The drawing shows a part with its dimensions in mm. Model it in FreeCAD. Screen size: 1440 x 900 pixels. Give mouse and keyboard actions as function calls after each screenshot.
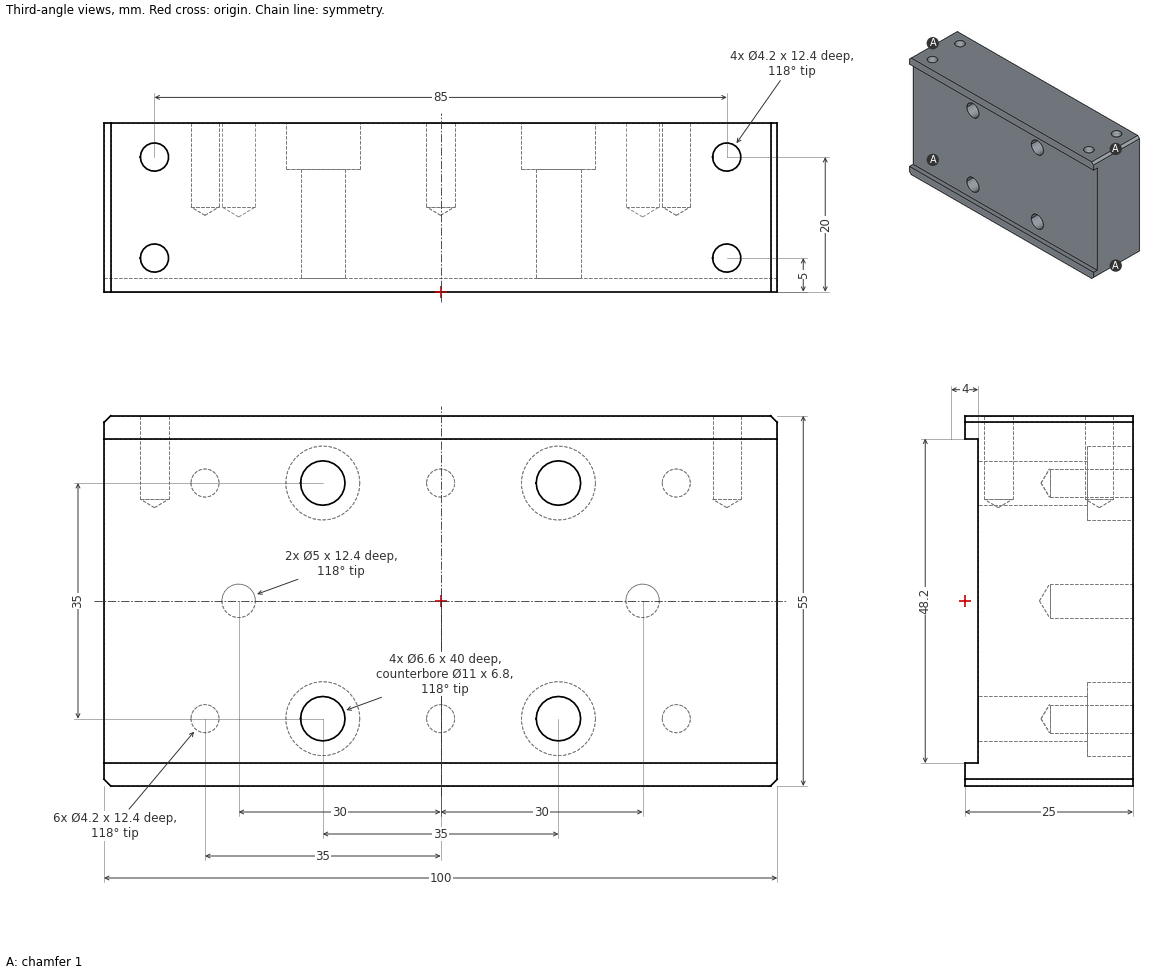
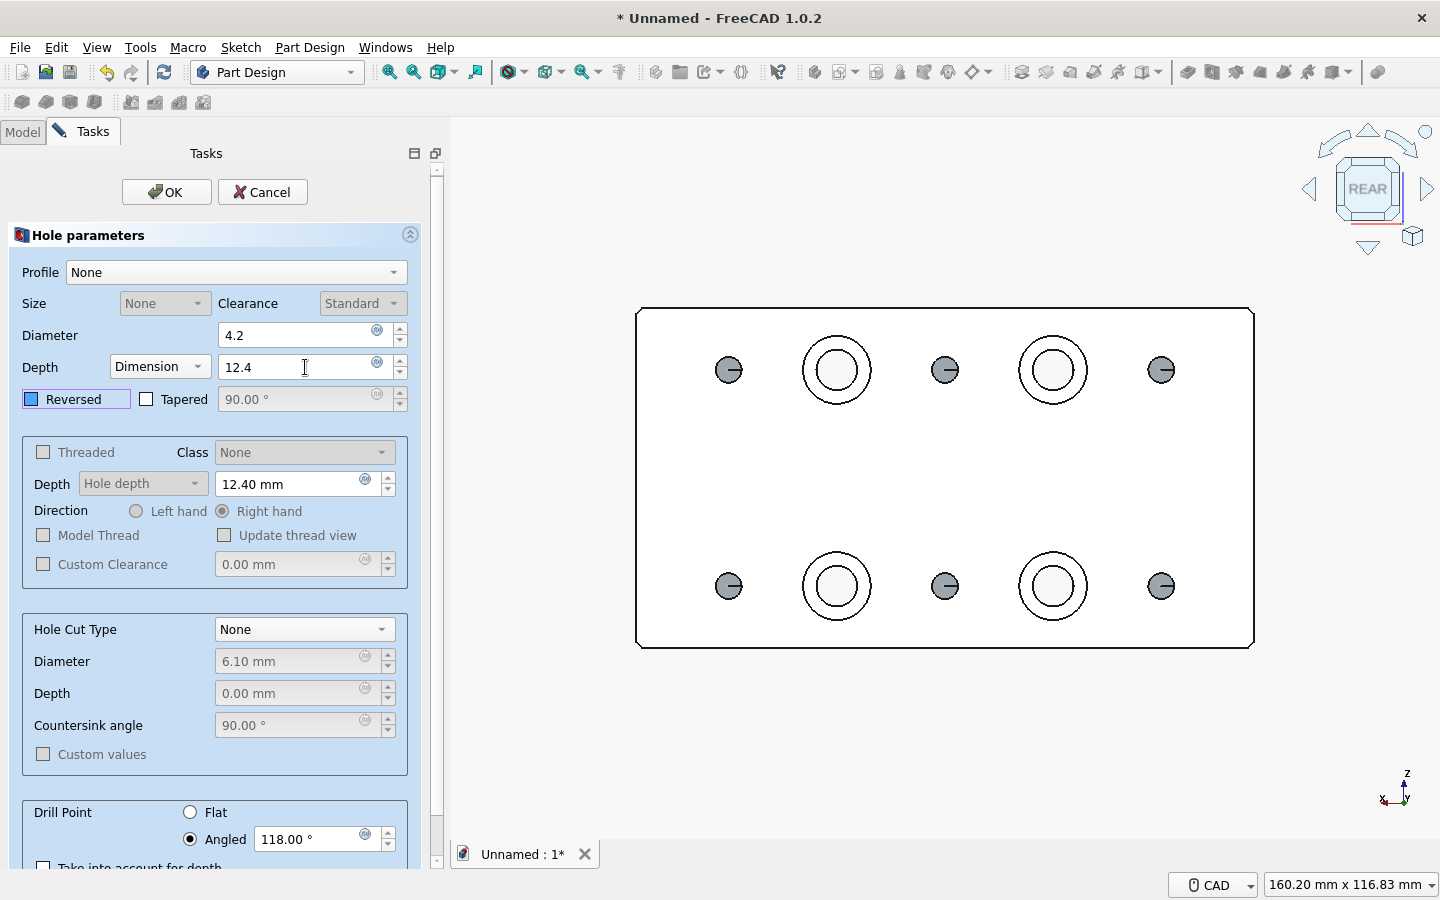
click(167, 192)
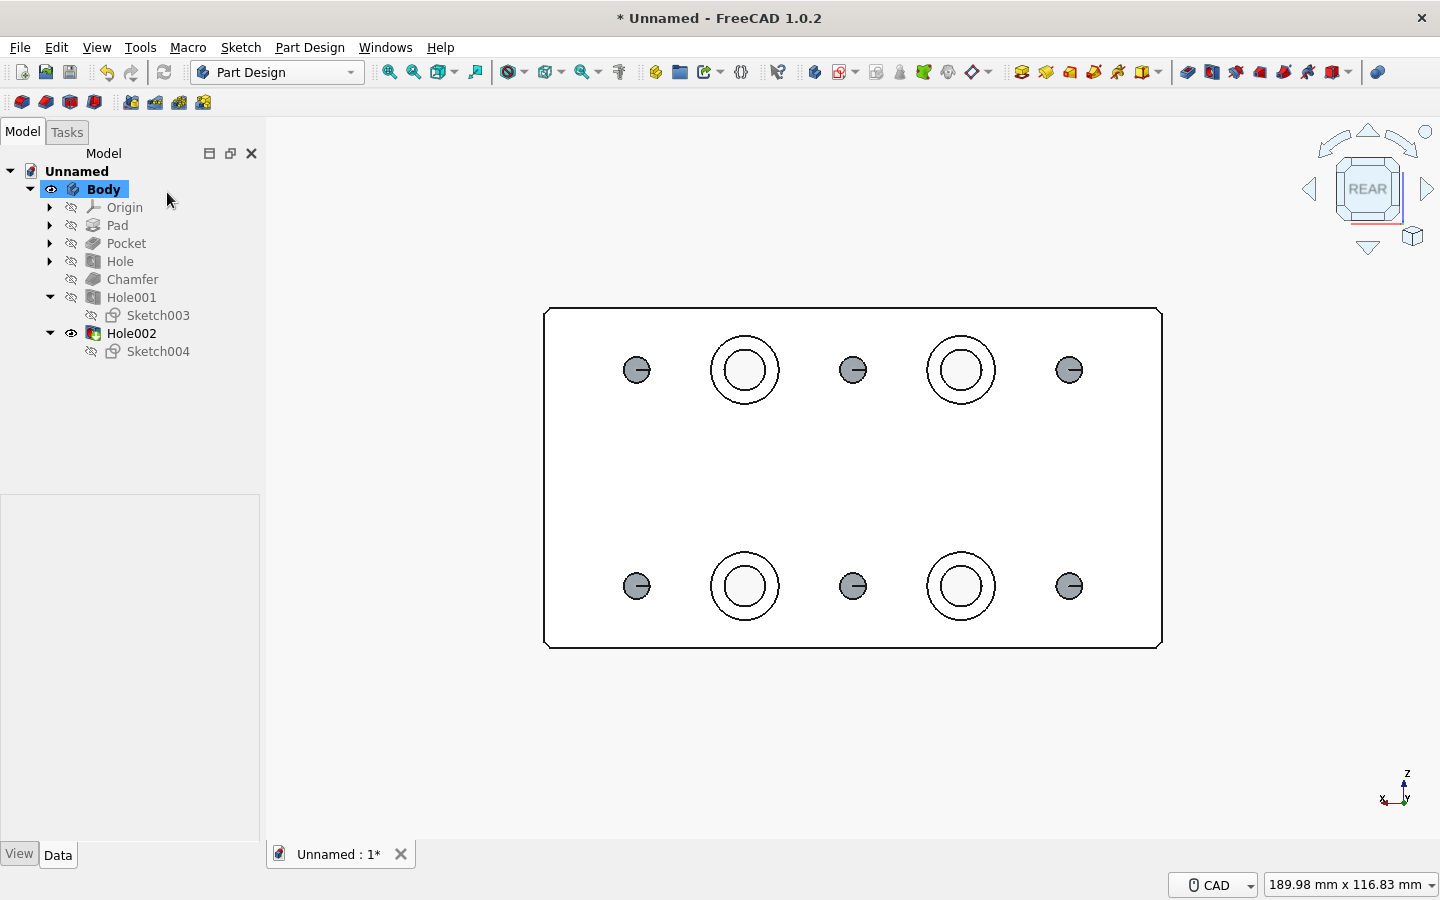
click(853, 477)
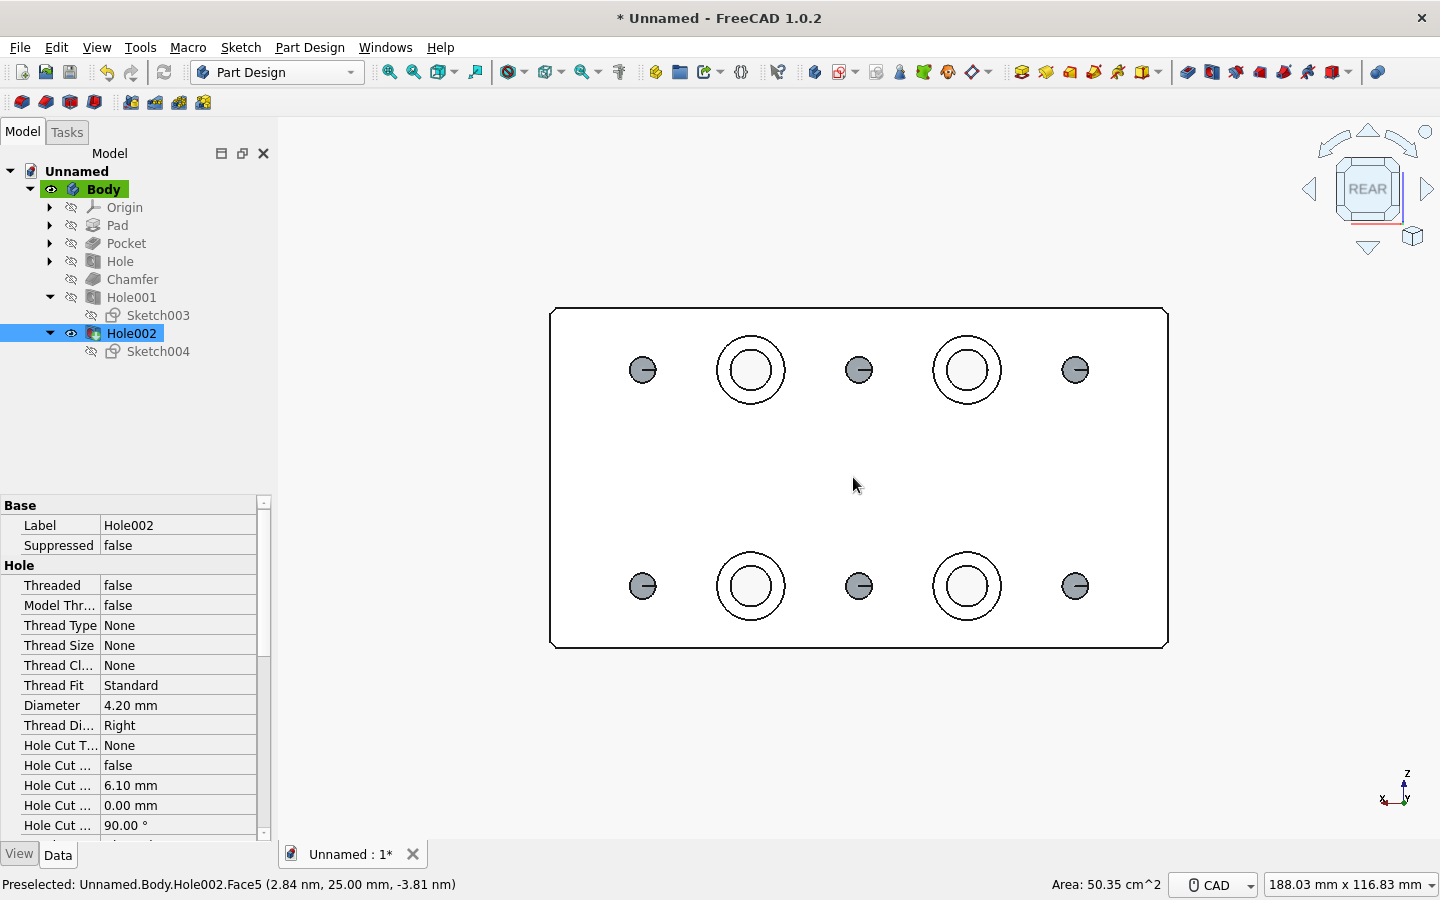
click(840, 72)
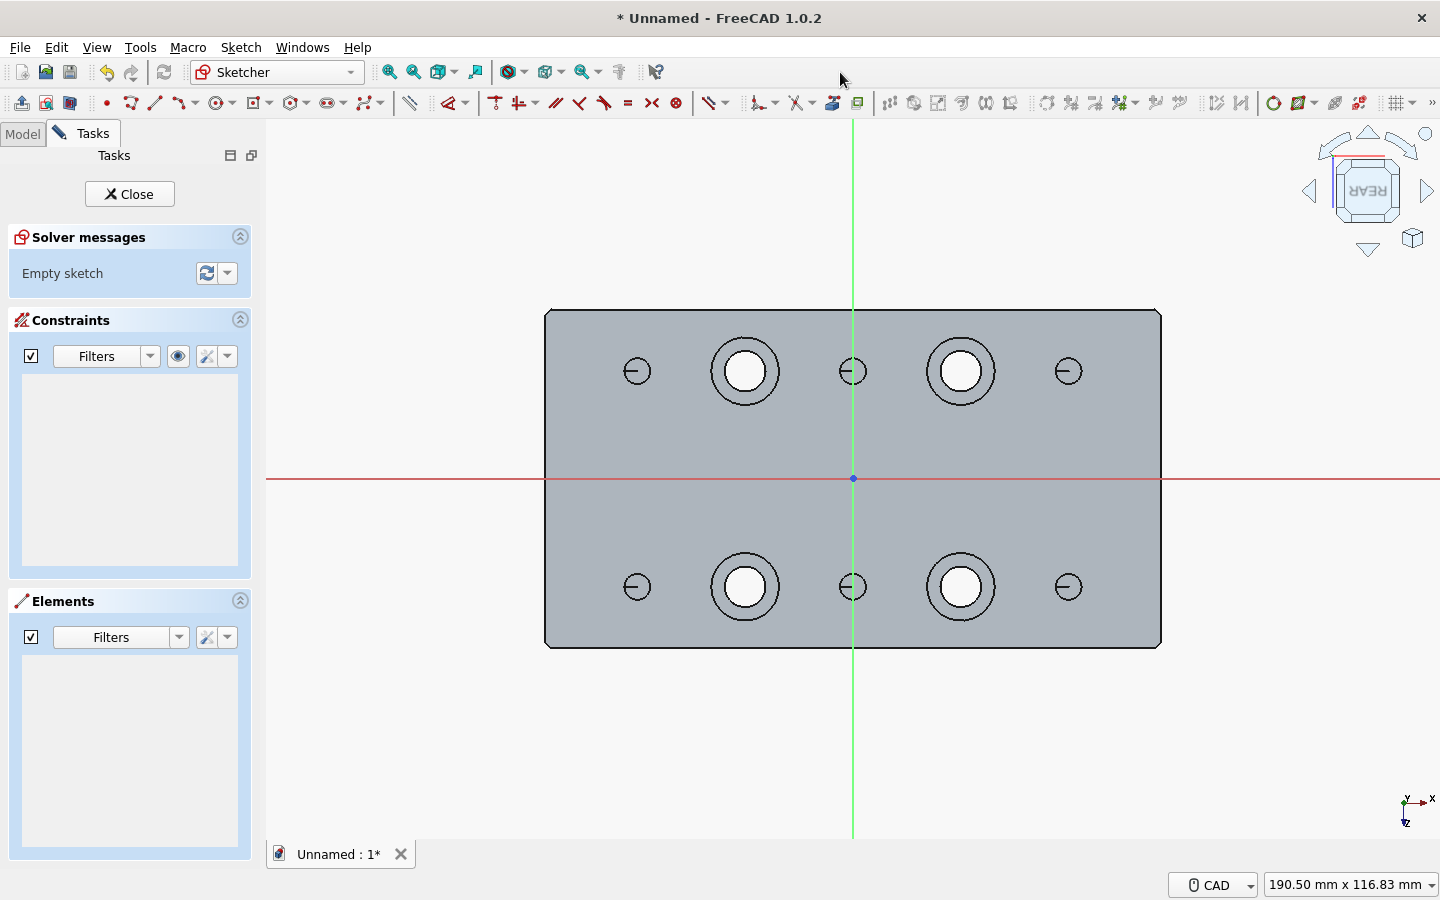
scroll(936, 479, up, 3)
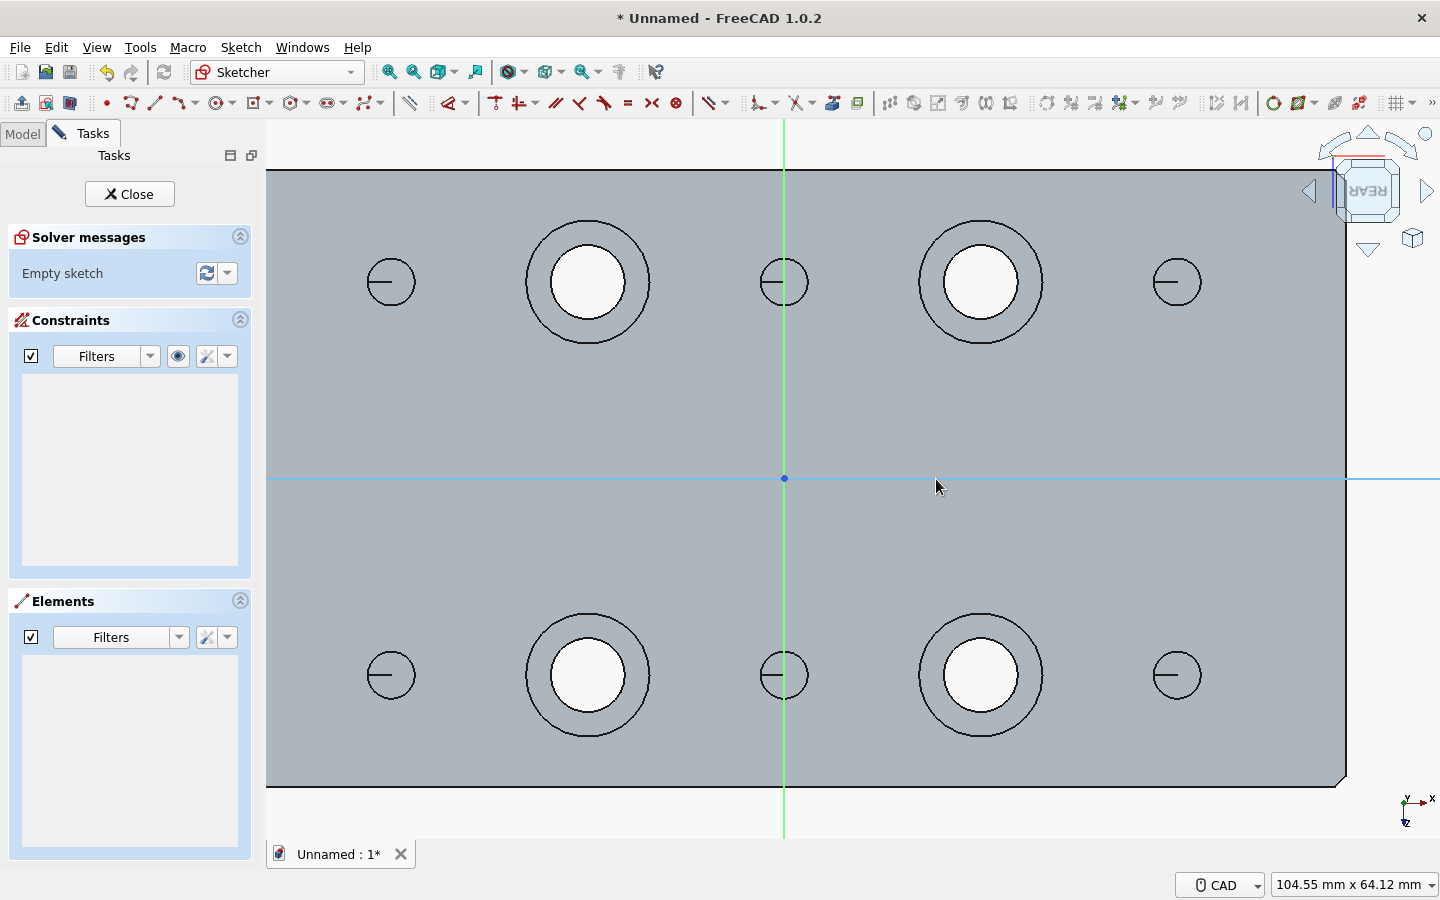
click(216, 104)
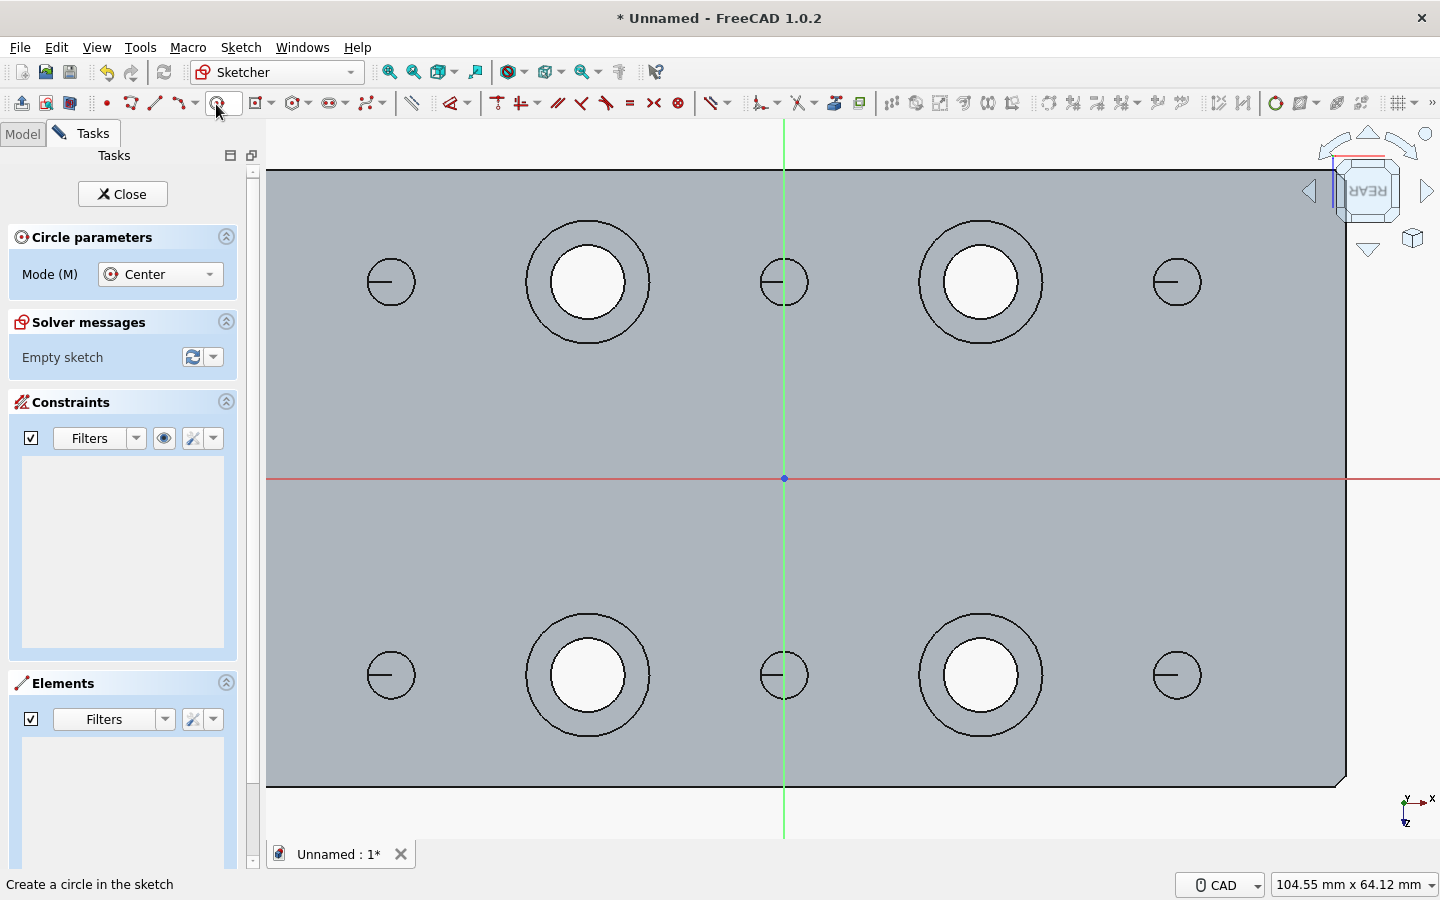
click(447, 479)
move(467, 459)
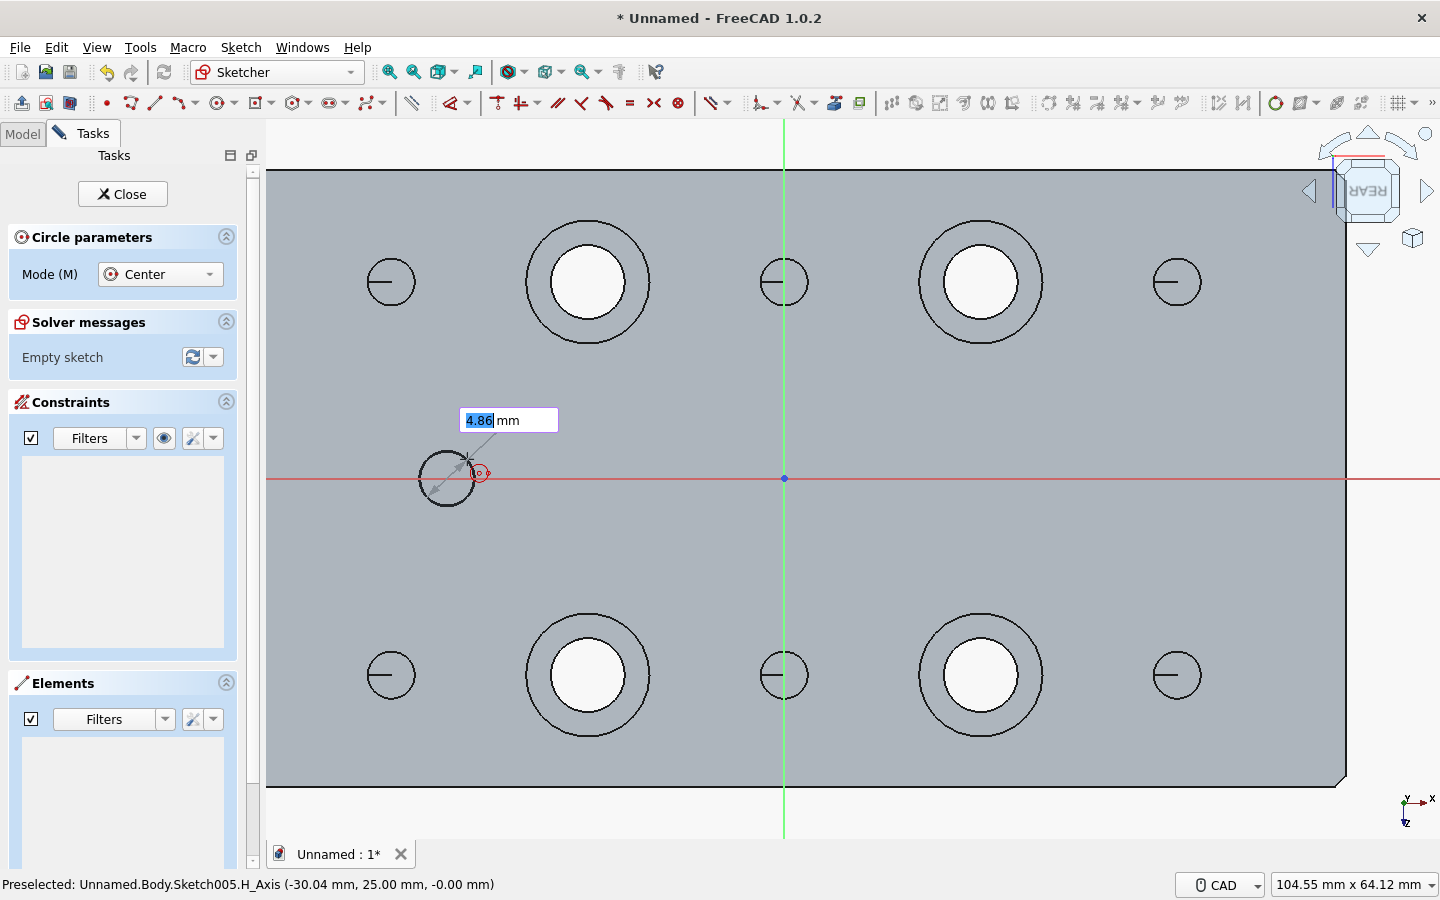
text(5)
key(Return)